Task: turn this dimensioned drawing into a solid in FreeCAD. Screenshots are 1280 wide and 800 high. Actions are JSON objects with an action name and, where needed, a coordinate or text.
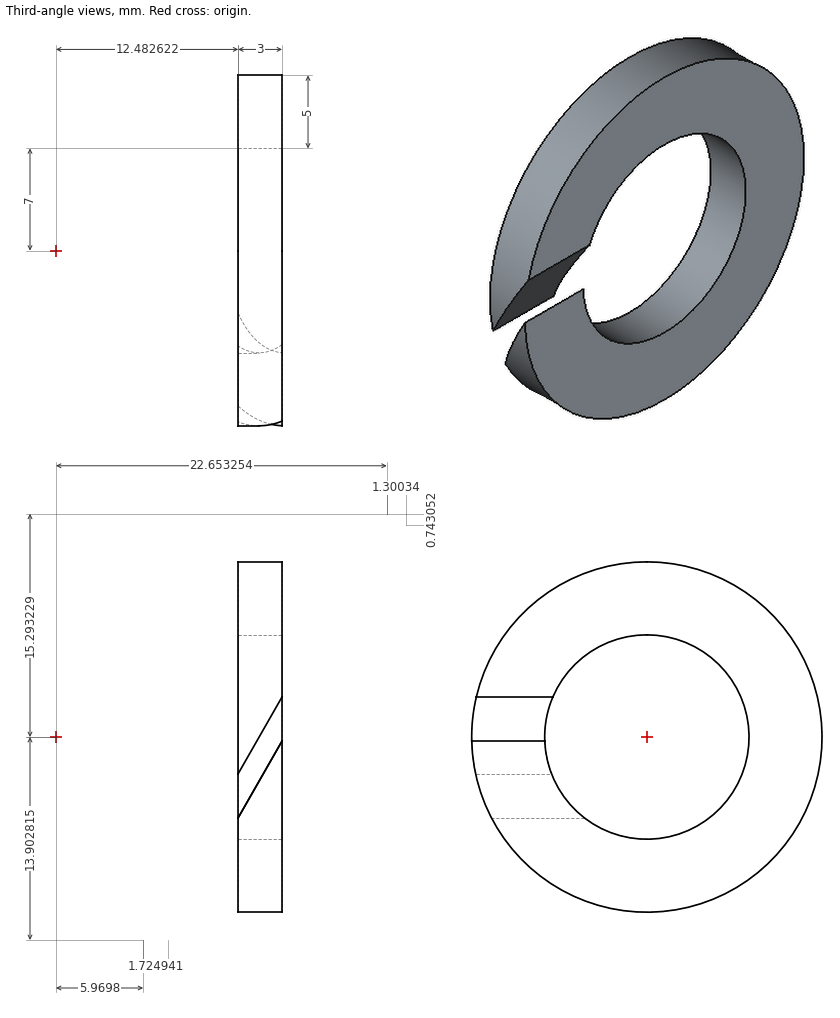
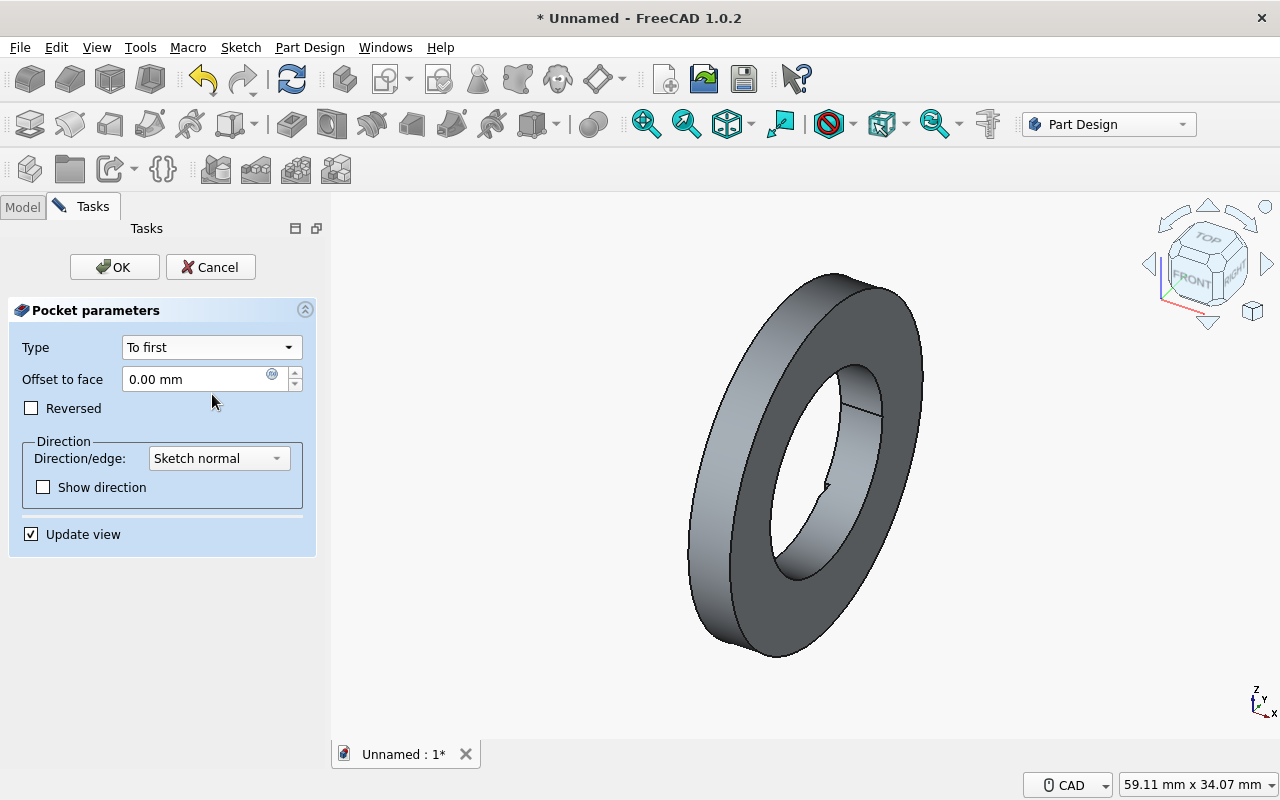
{"action": "left_click", "coordinate": [30, 408]}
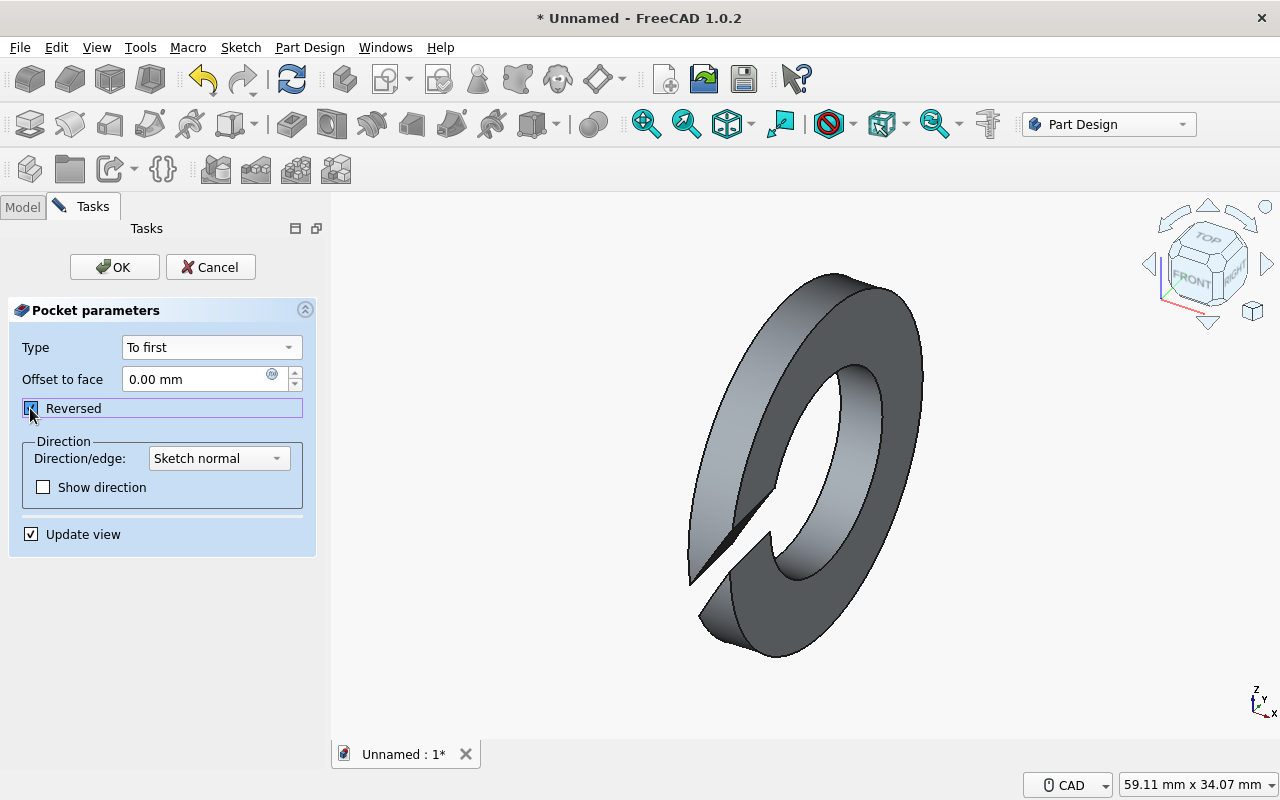
{"action": "left_click", "coordinate": [115, 267]}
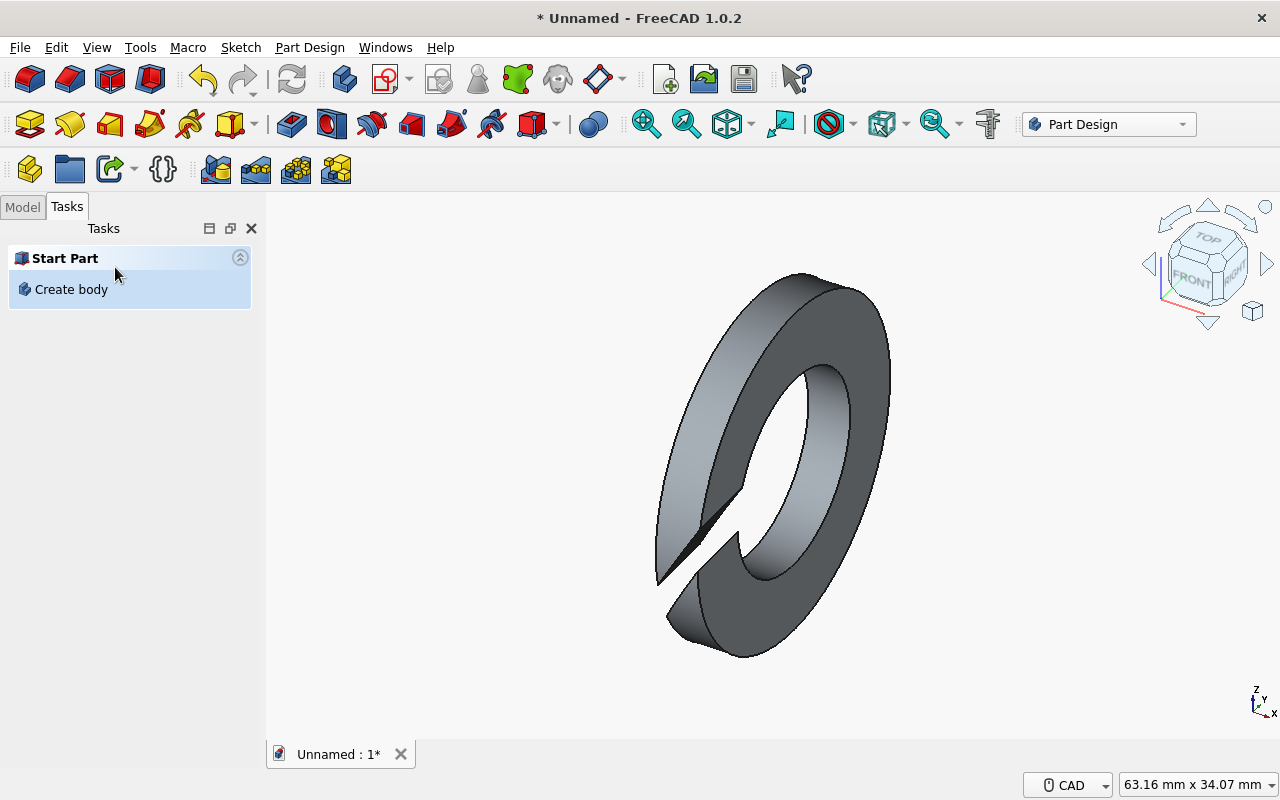
{"action": "key", "text": "0"}